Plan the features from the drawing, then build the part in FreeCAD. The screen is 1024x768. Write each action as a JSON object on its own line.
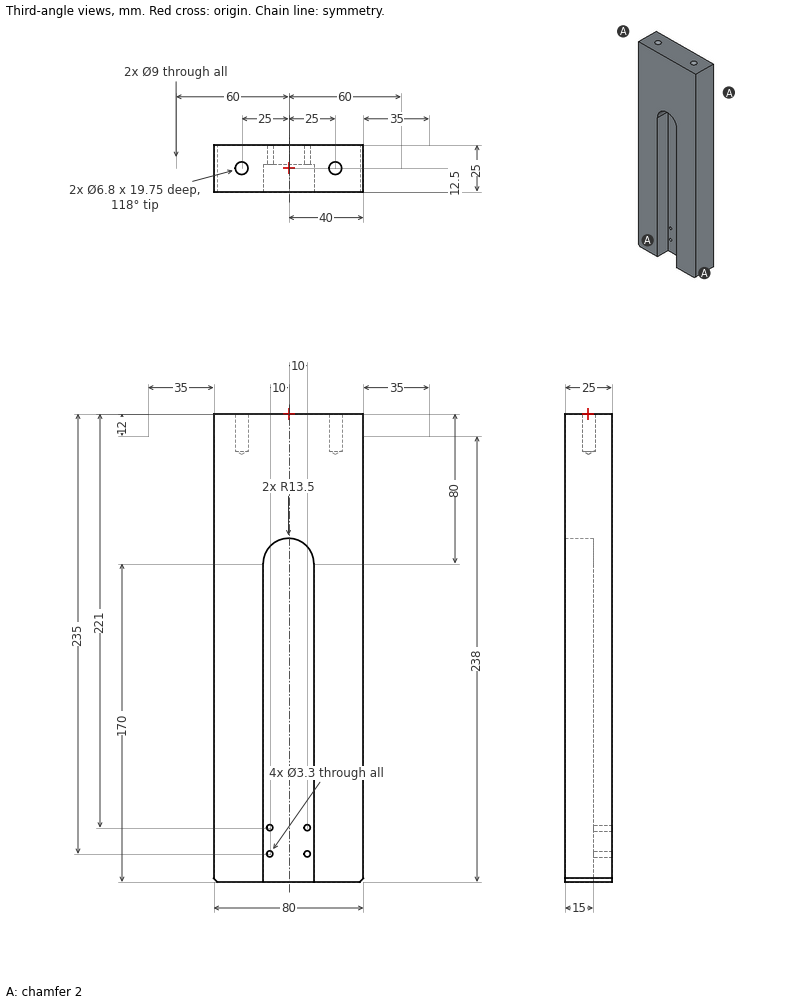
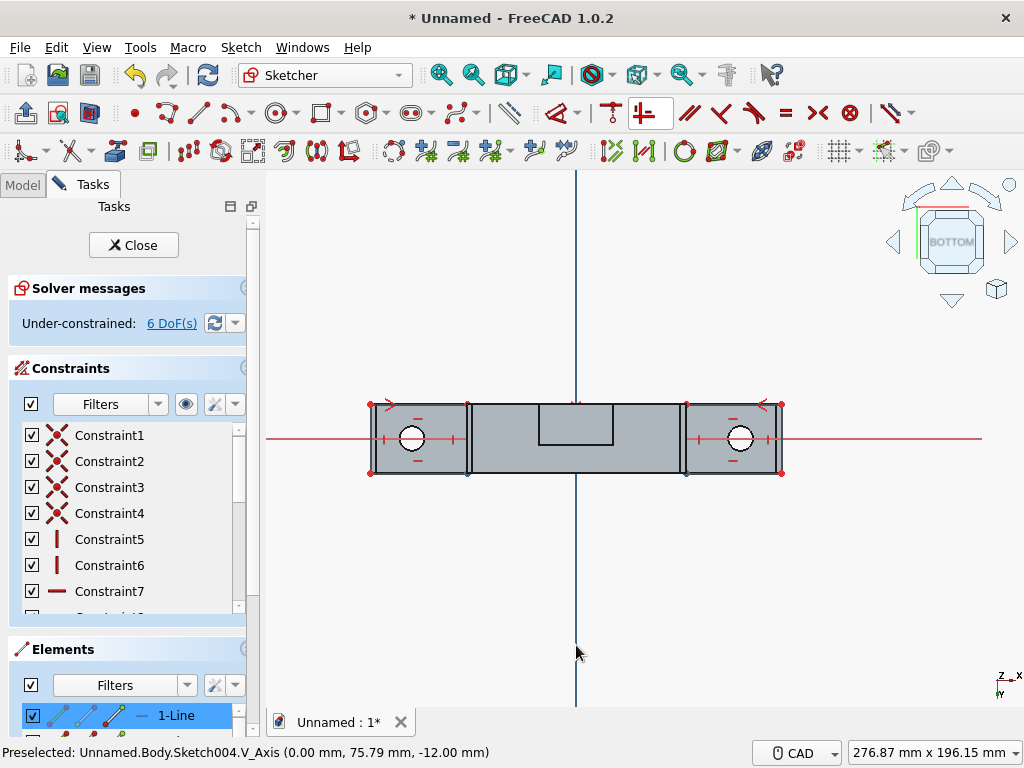
{"action": "left_click", "coordinate": [818, 114]}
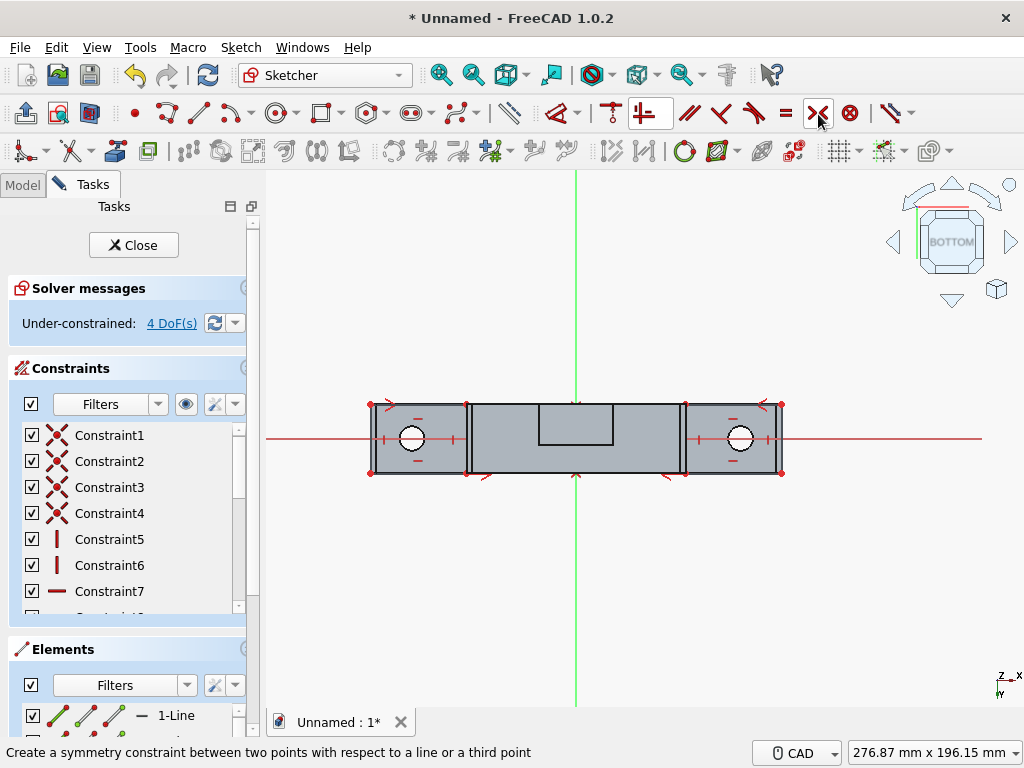
{"action": "left_click", "coordinate": [556, 114]}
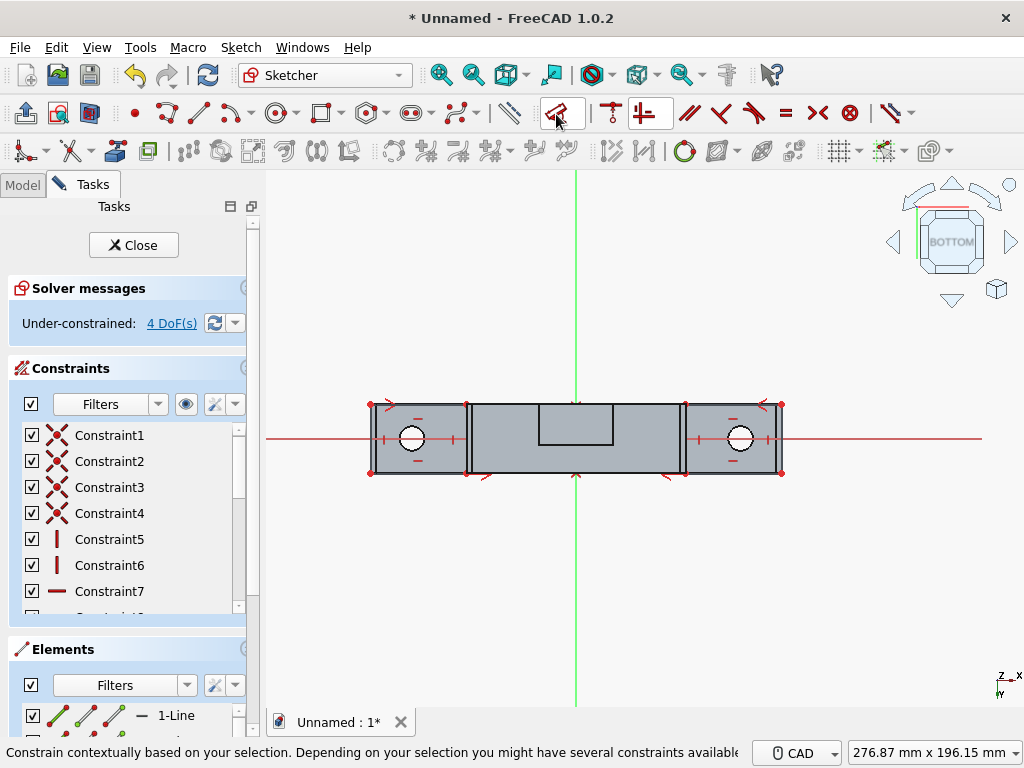
{"action": "left_click", "coordinate": [686, 426]}
{"action": "left_click", "coordinate": [720, 424]}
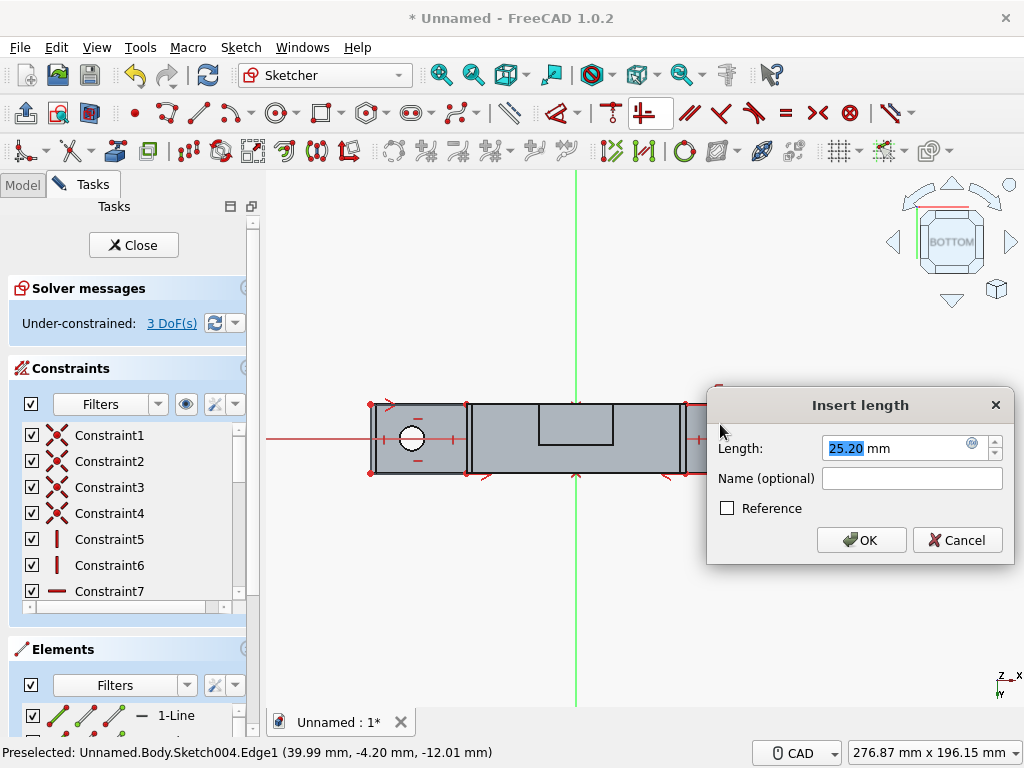
{"action": "type", "text": "25"}
{"action": "key", "text": "Return"}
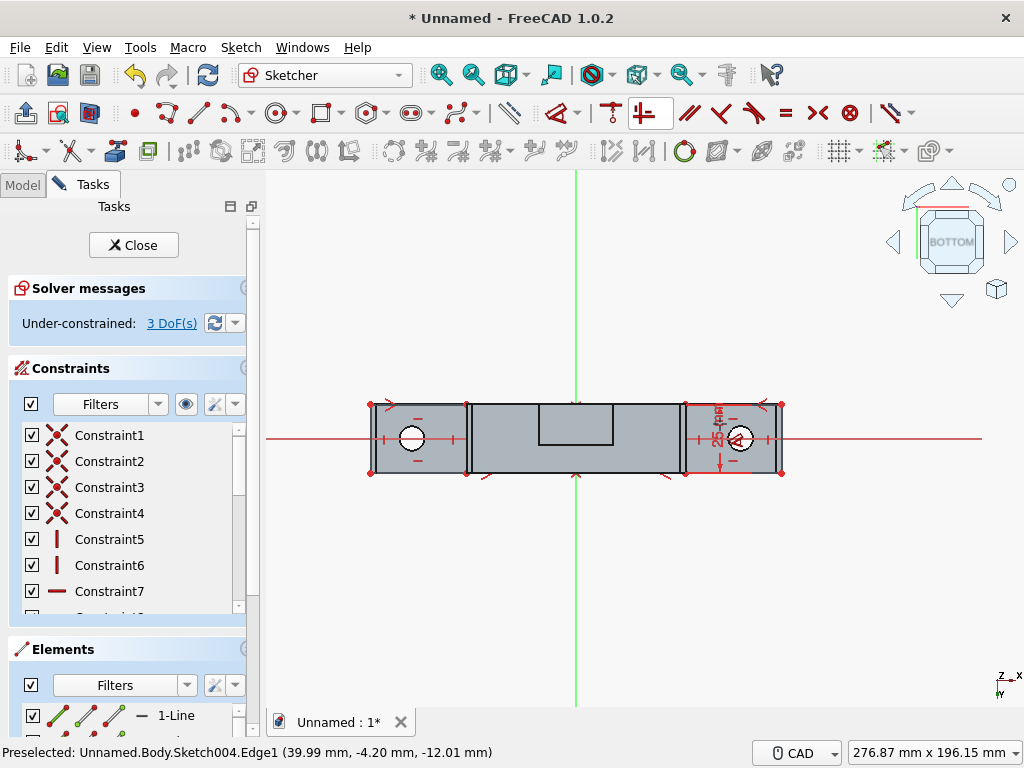
{"action": "left_click", "coordinate": [715, 473]}
{"action": "left_click", "coordinate": [734, 507]}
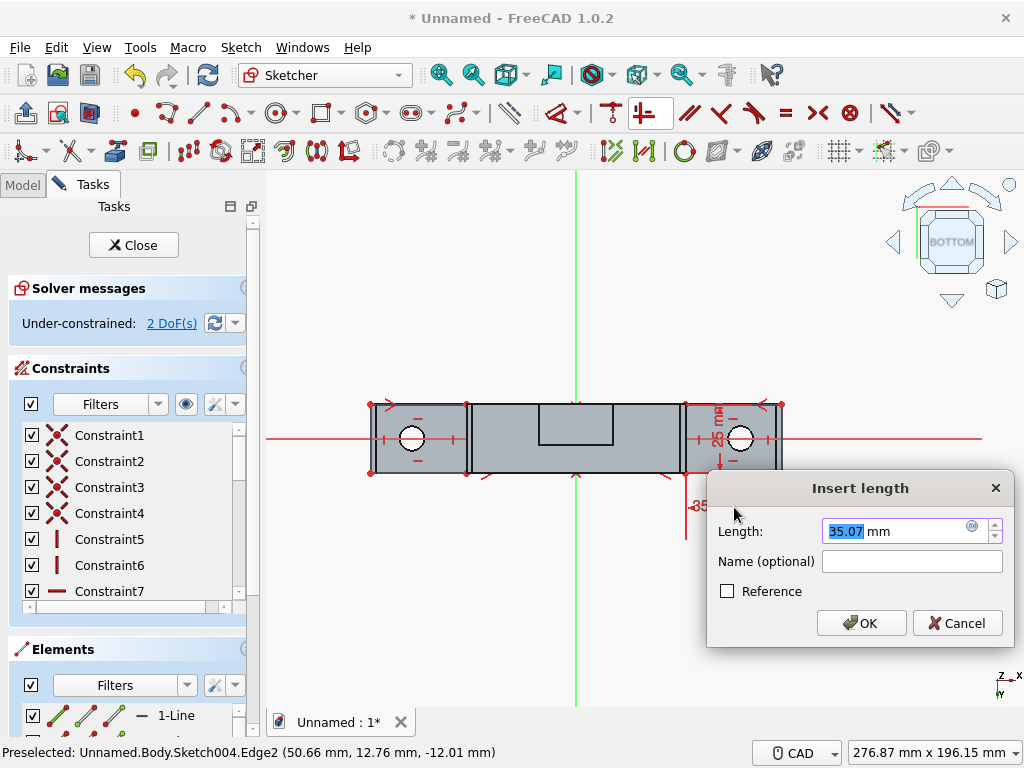
{"action": "type", "text": "35"}
{"action": "key", "text": "Return"}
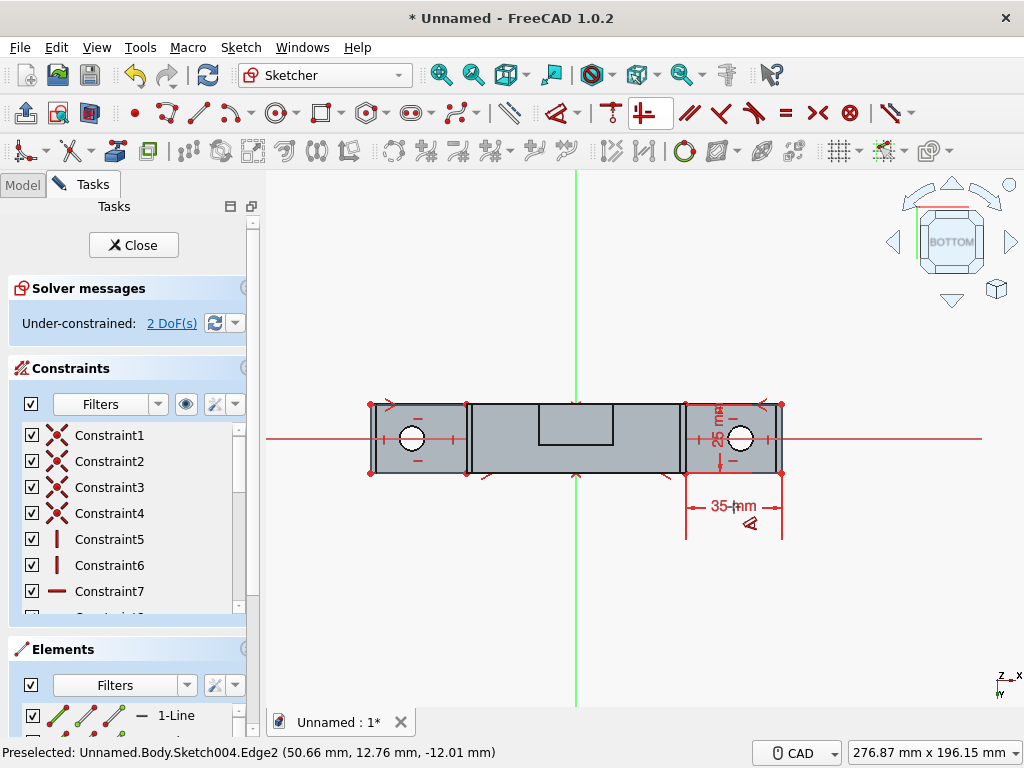
{"action": "left_click", "coordinate": [686, 405]}
{"action": "left_click", "coordinate": [631, 371]}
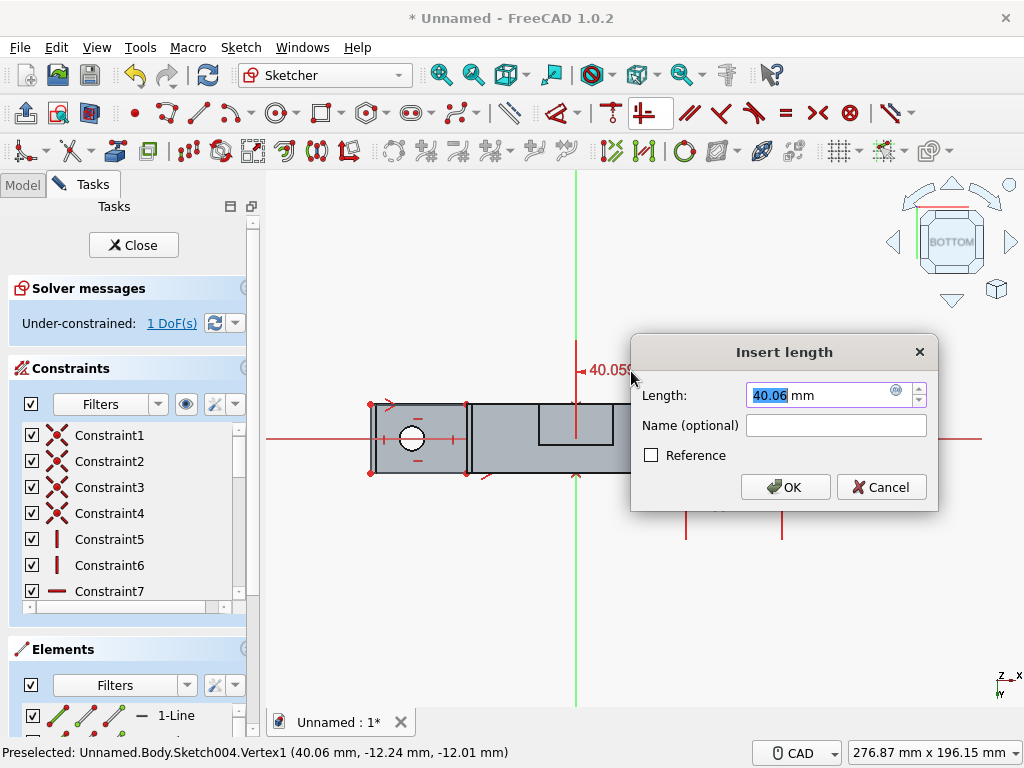
{"action": "type", "text": "40"}
{"action": "key", "text": "Return"}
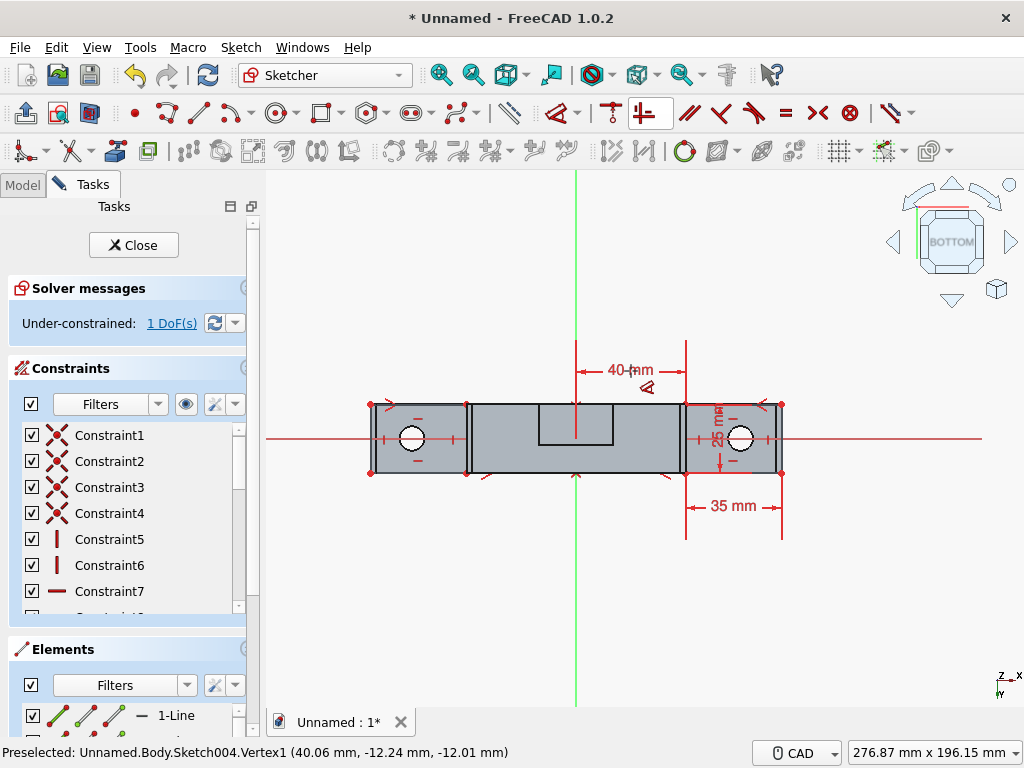
{"action": "left_click", "coordinate": [686, 405]}
{"action": "left_click", "coordinate": [542, 422]}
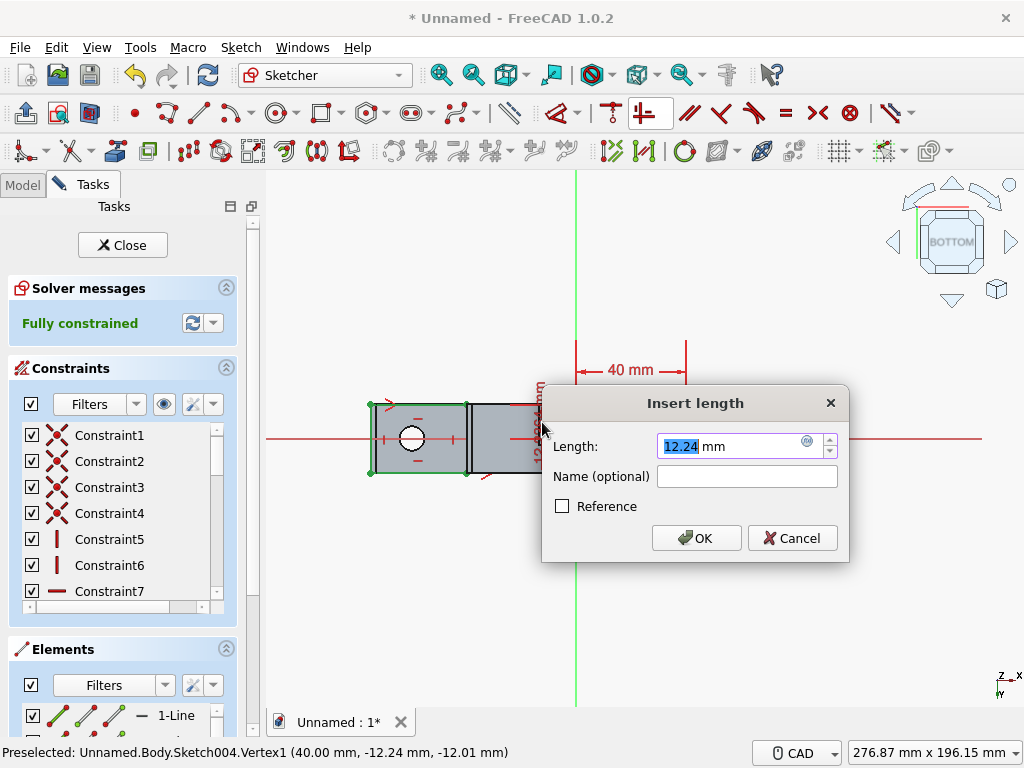
{"action": "type", "text": "12.5"}
{"action": "key", "text": "Return"}
{"action": "key", "text": "Escape"}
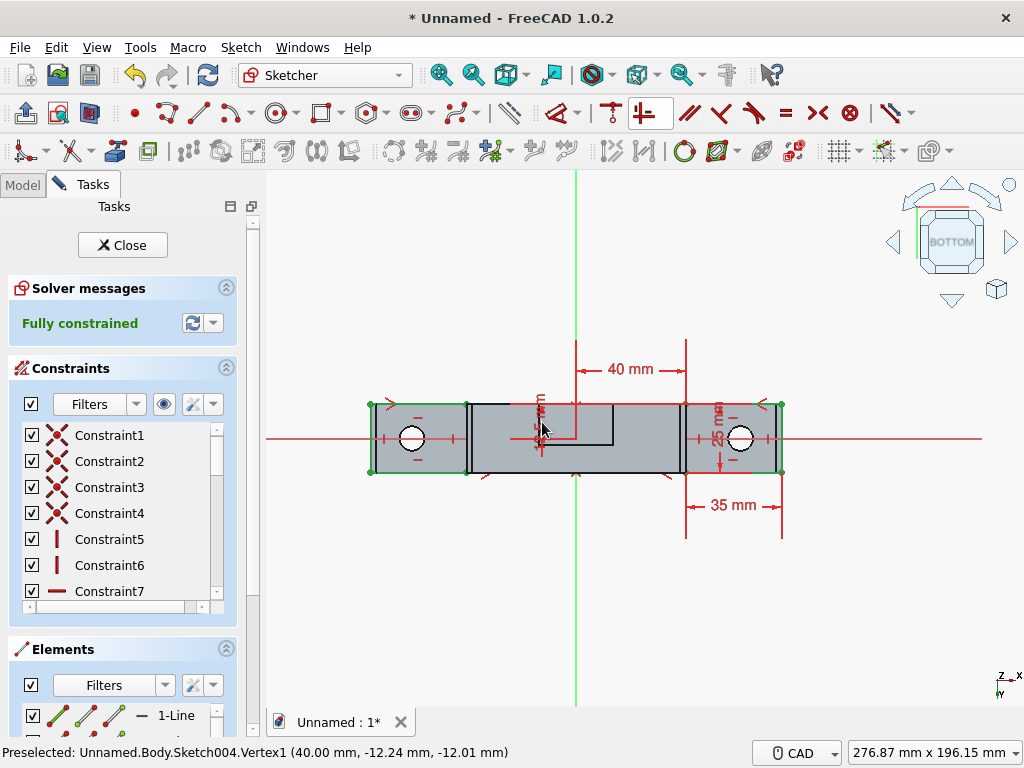
{"action": "left_click", "coordinate": [123, 245]}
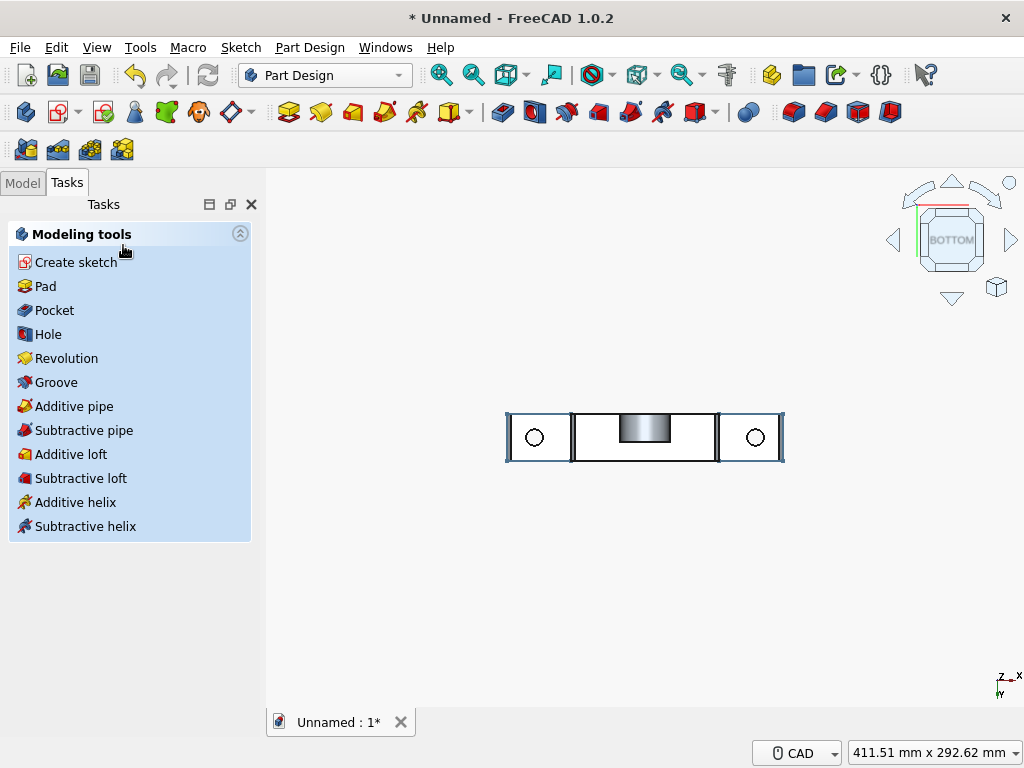
{"action": "left_click", "coordinate": [504, 112]}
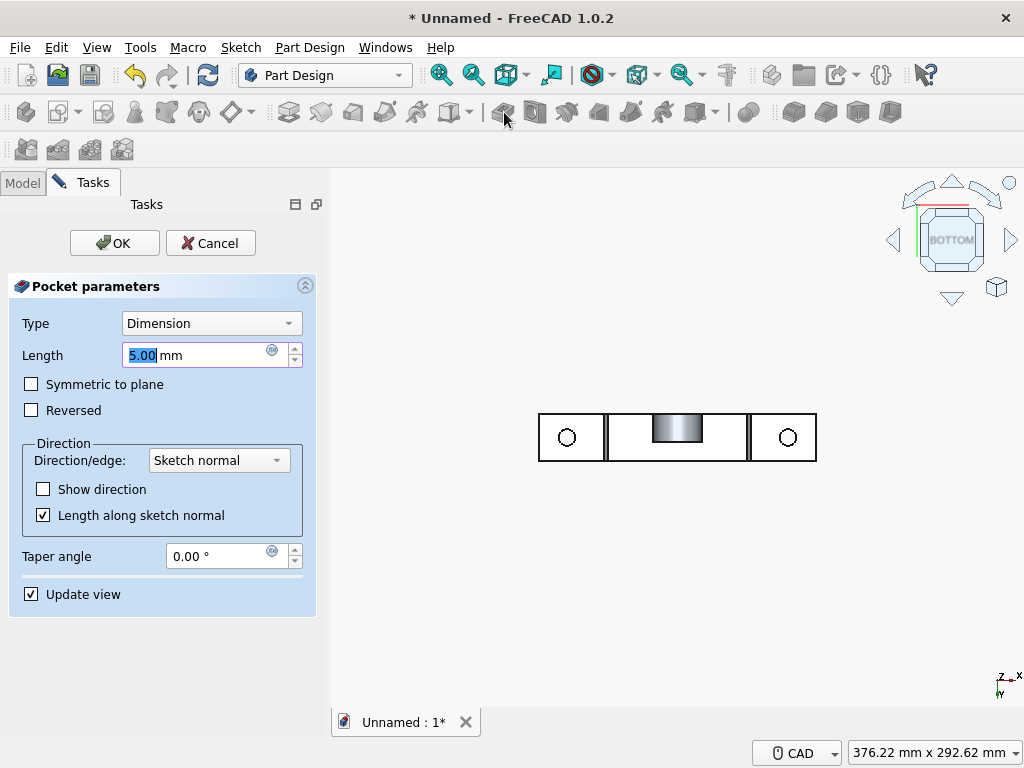
{"action": "left_click", "coordinate": [212, 324]}